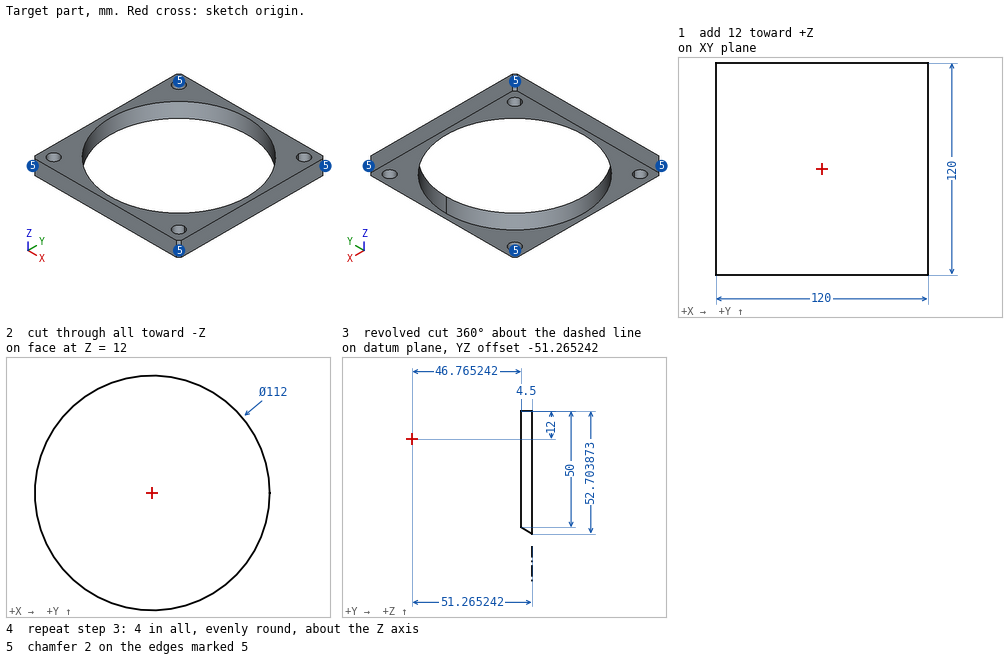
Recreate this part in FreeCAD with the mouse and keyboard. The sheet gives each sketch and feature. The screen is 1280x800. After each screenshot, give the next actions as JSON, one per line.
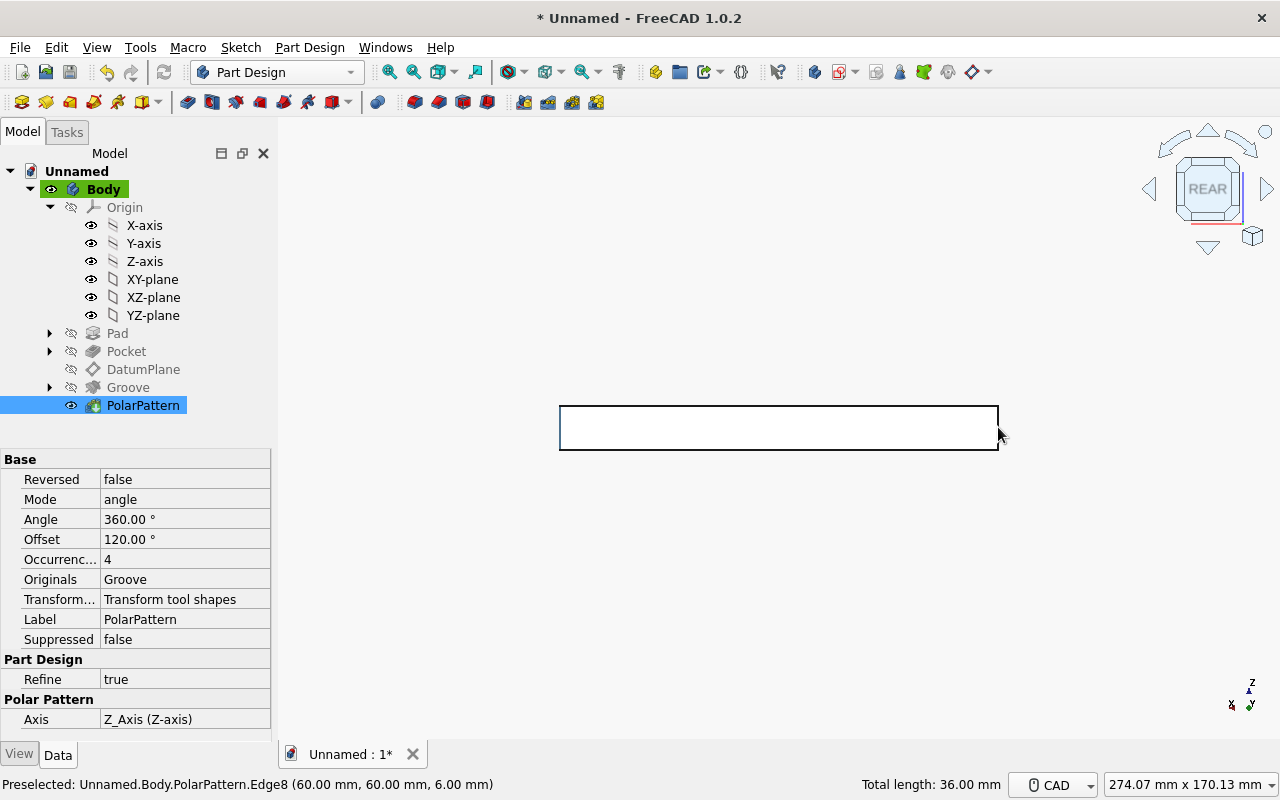
{"action": "key", "text": "v f"}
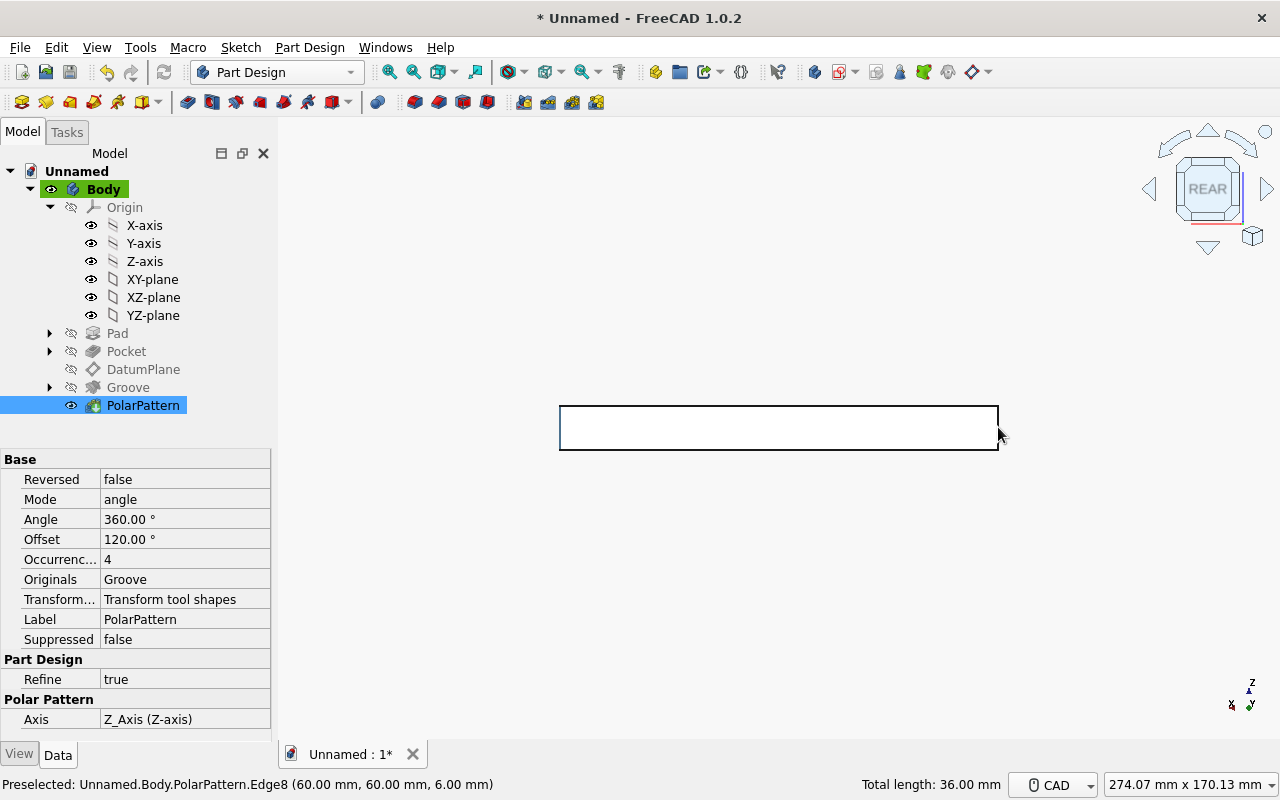
{"action": "left_click", "coordinate": [998, 427], "text": "ctrl"}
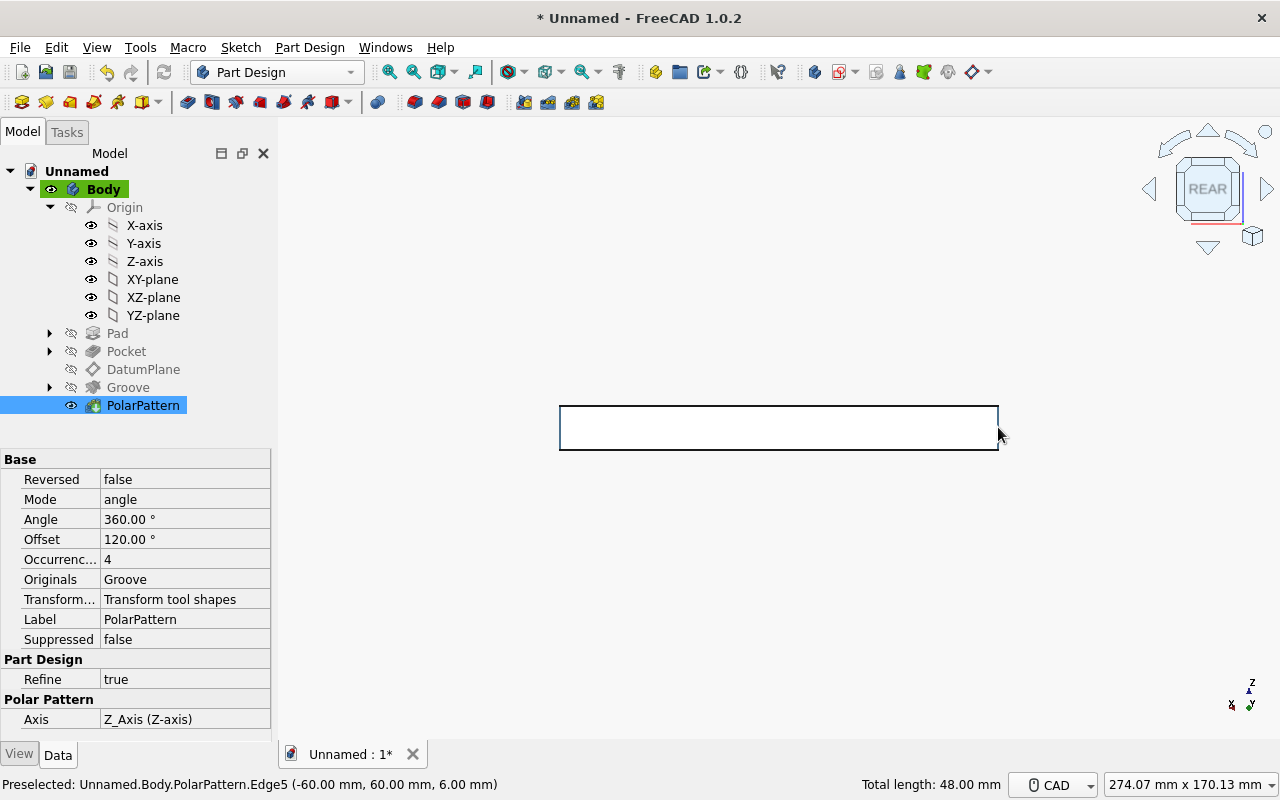
{"action": "left_click", "coordinate": [440, 102]}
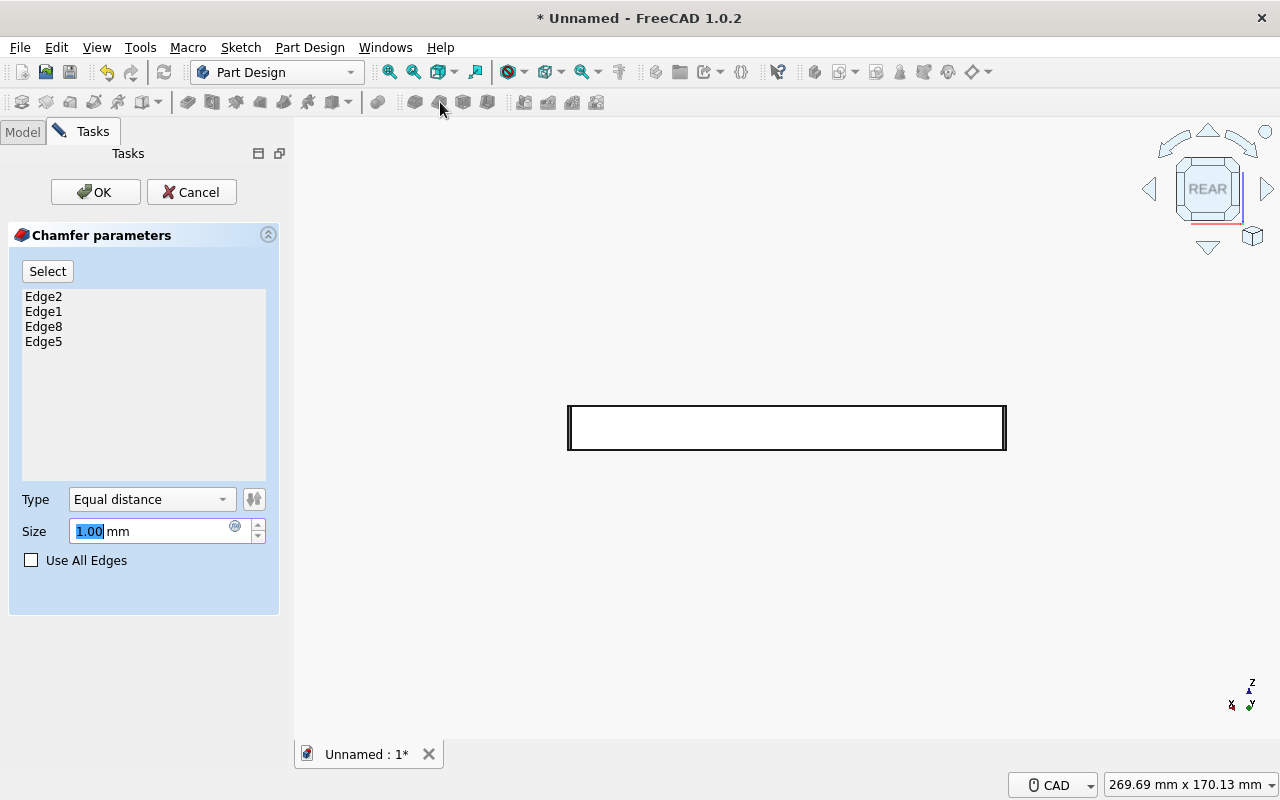
{"action": "type", "text": "2"}
{"action": "key", "text": "Tab"}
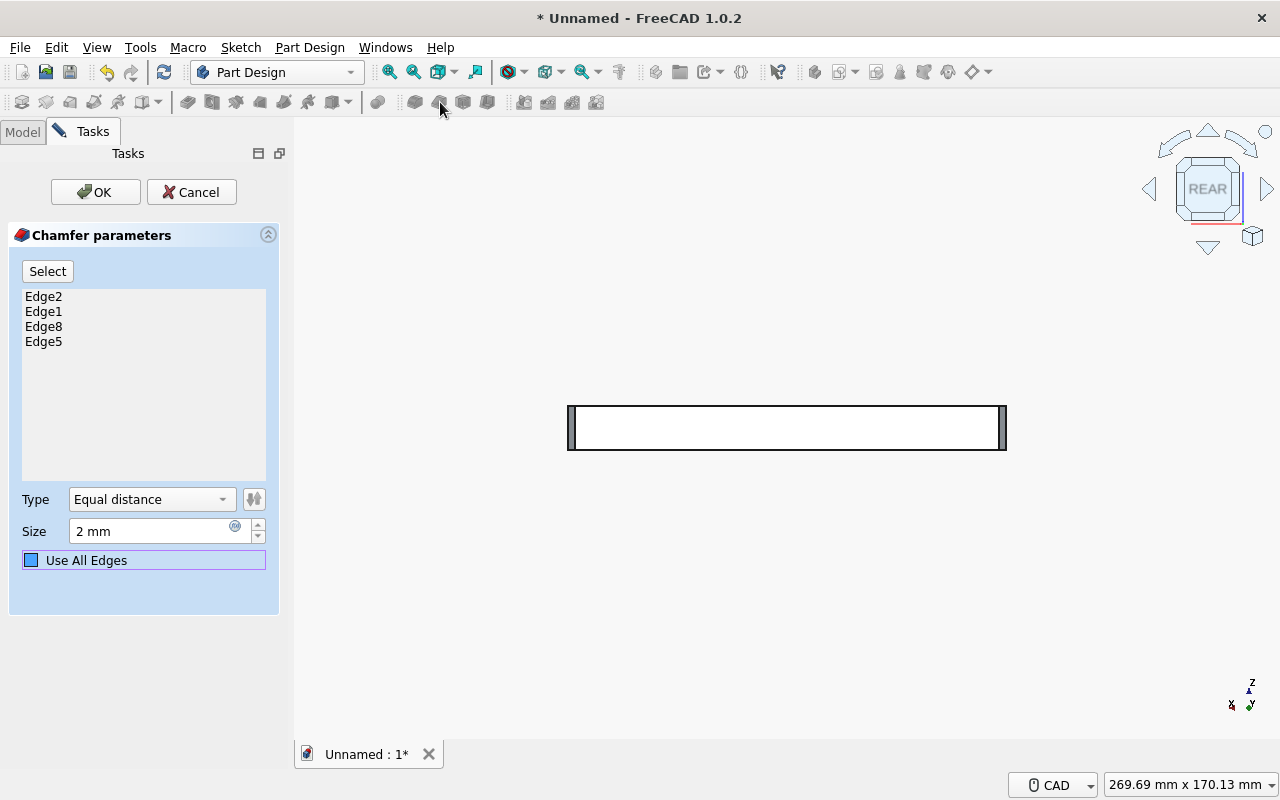
{"action": "left_click", "coordinate": [96, 192]}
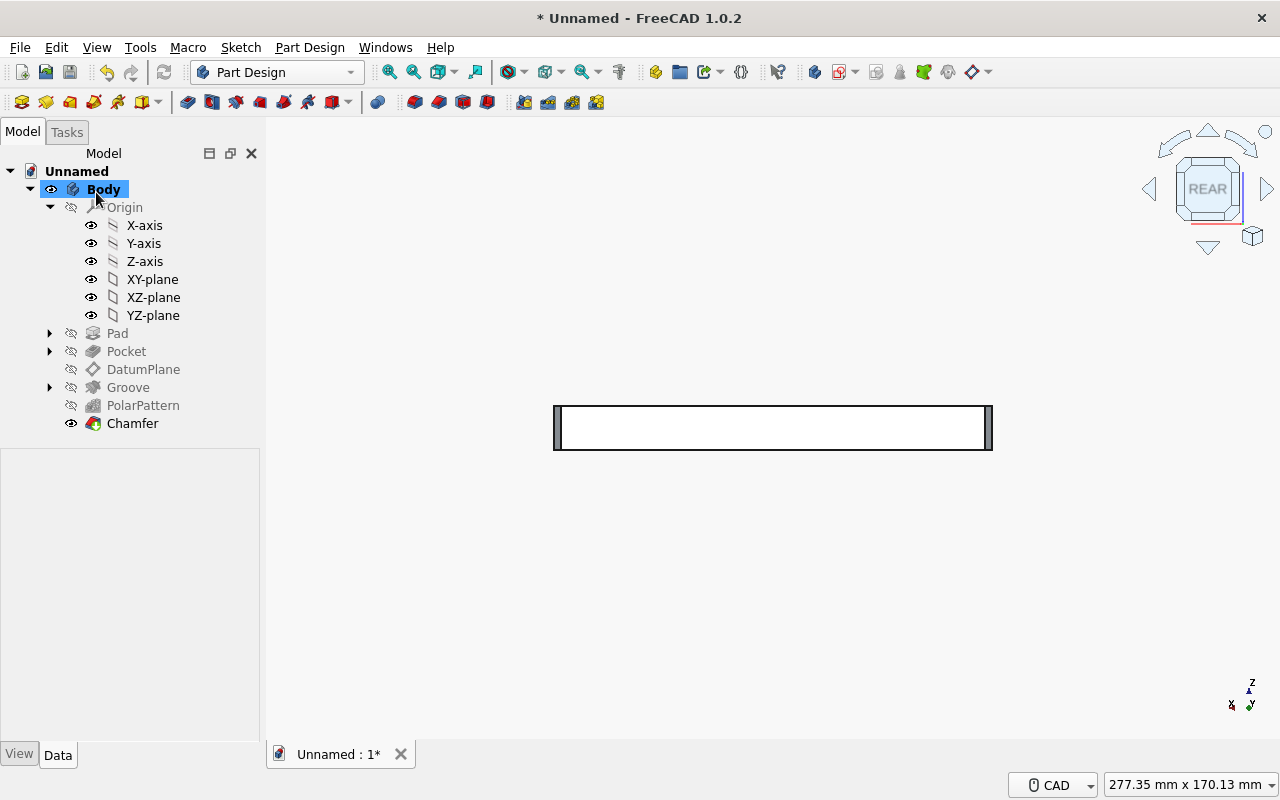
{"action": "key", "text": "0"}